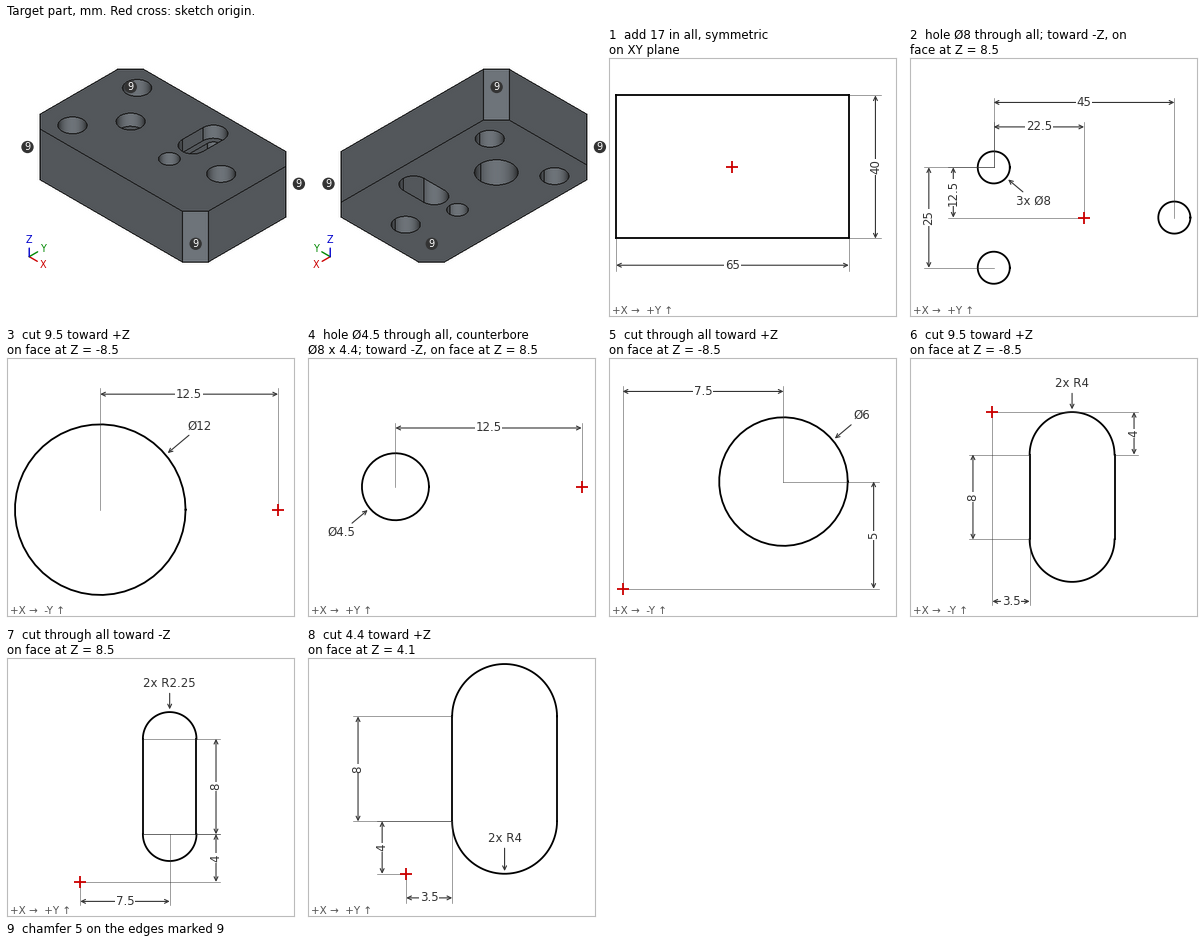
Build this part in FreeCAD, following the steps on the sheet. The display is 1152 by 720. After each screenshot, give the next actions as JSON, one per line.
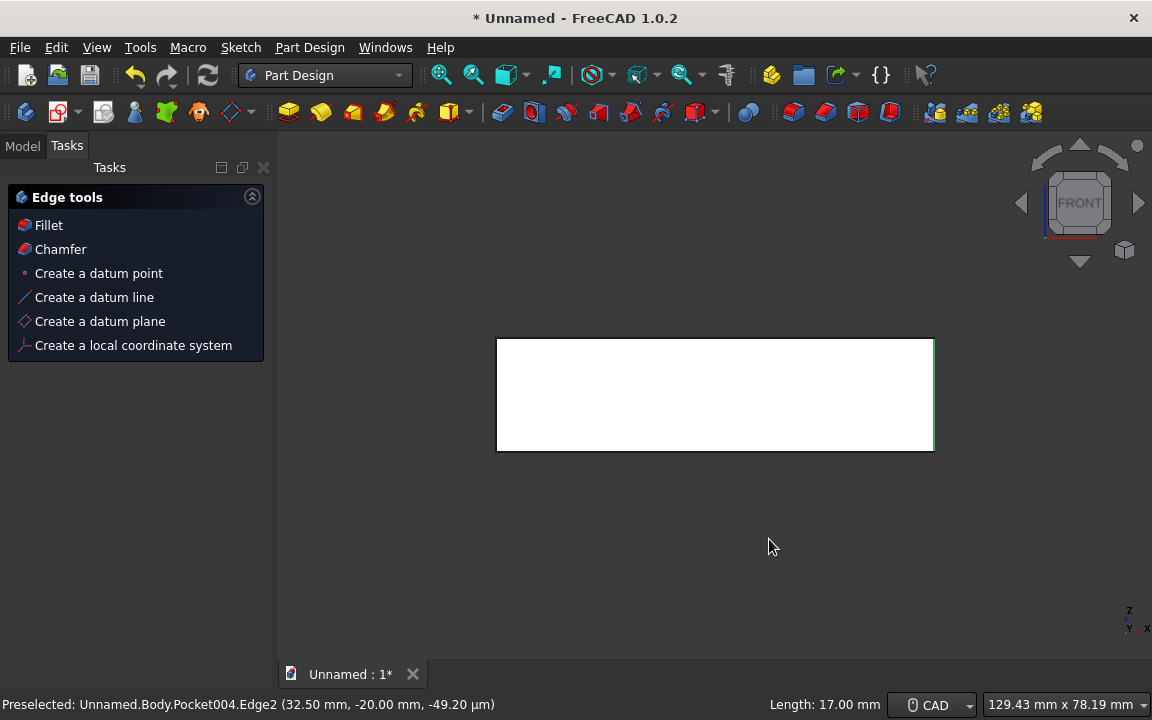
{"action": "left_click", "coordinate": [496, 394], "text": "ctrl"}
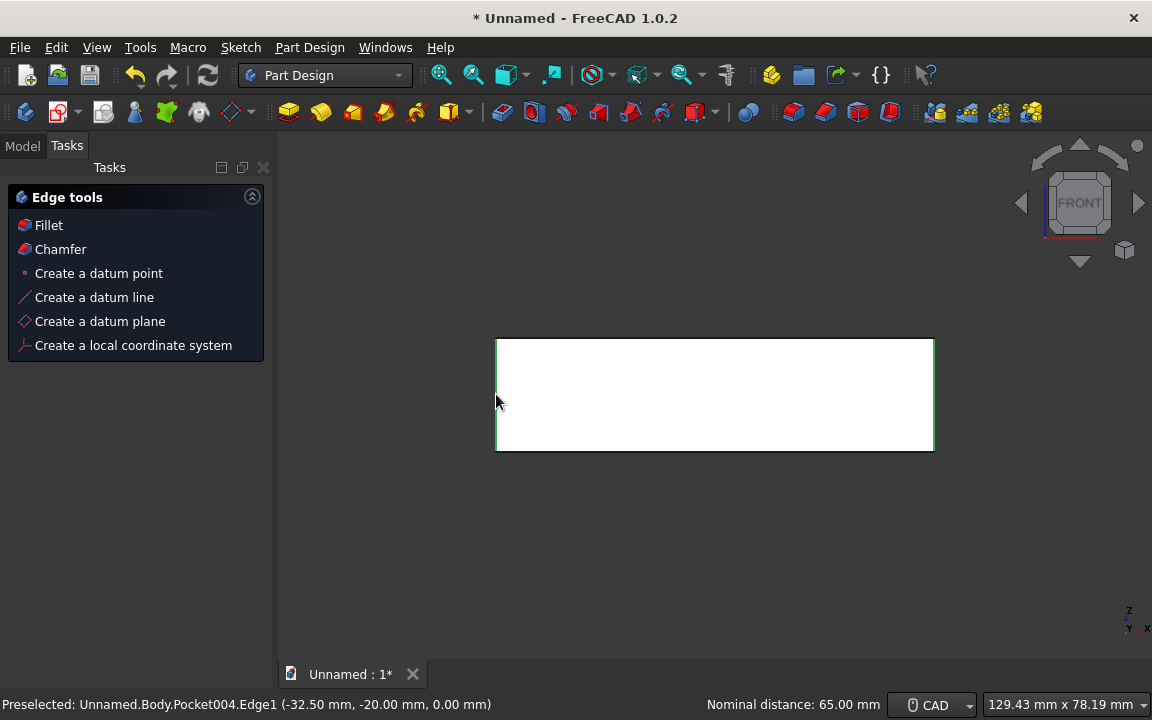
{"action": "key", "text": "3"}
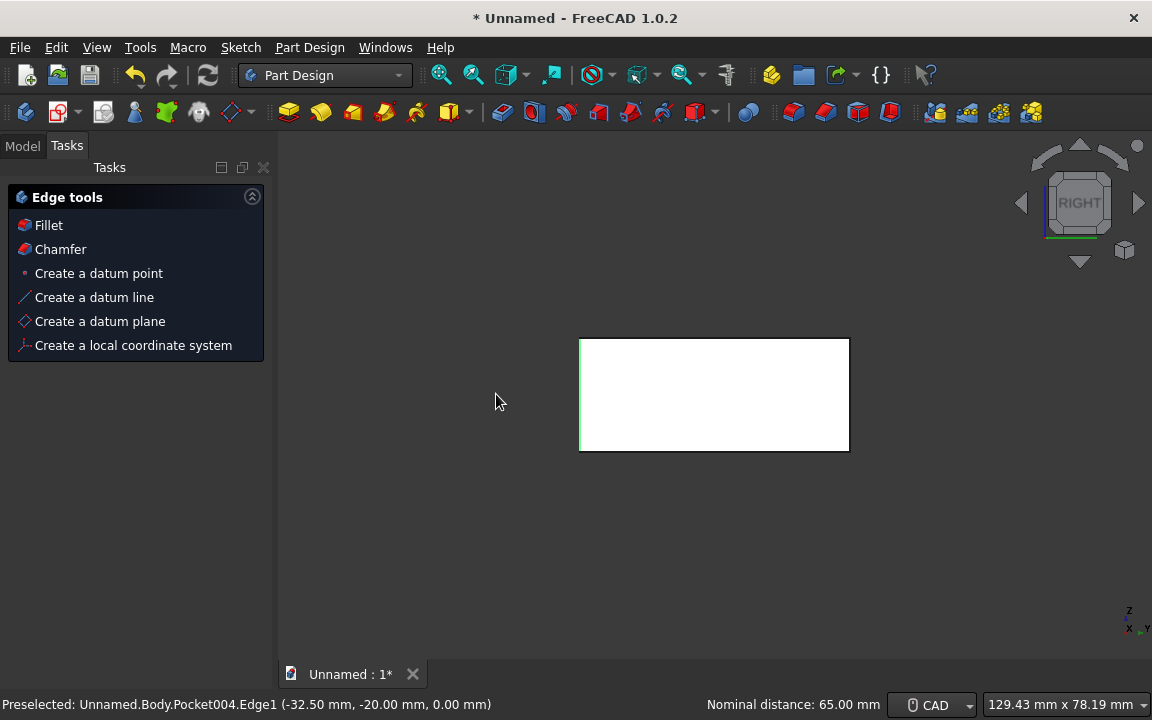
{"action": "left_click", "coordinate": [442, 76]}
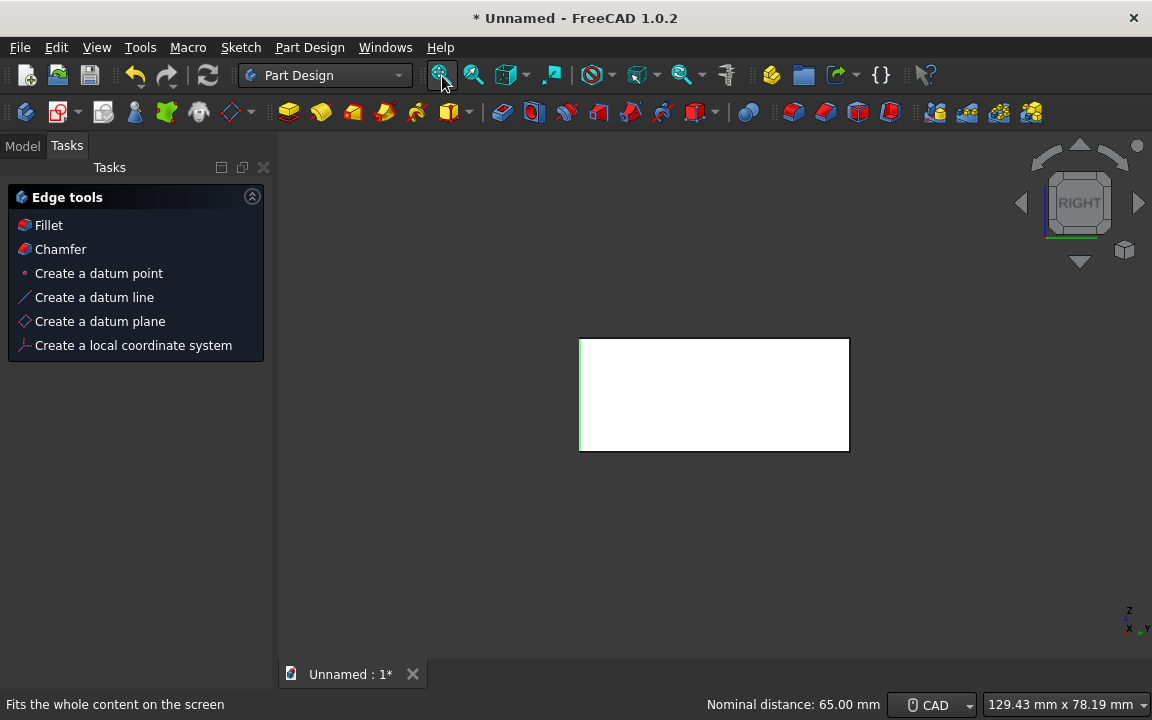
{"action": "left_click", "coordinate": [850, 394], "text": "ctrl"}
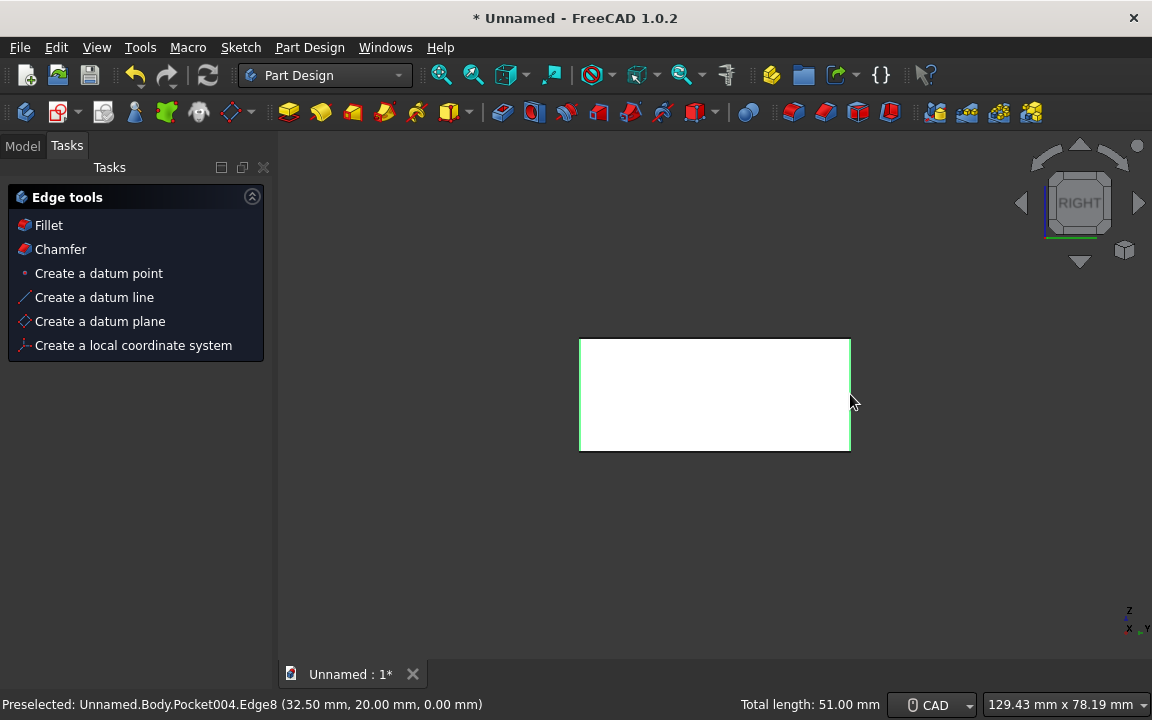
{"action": "key", "text": "5"}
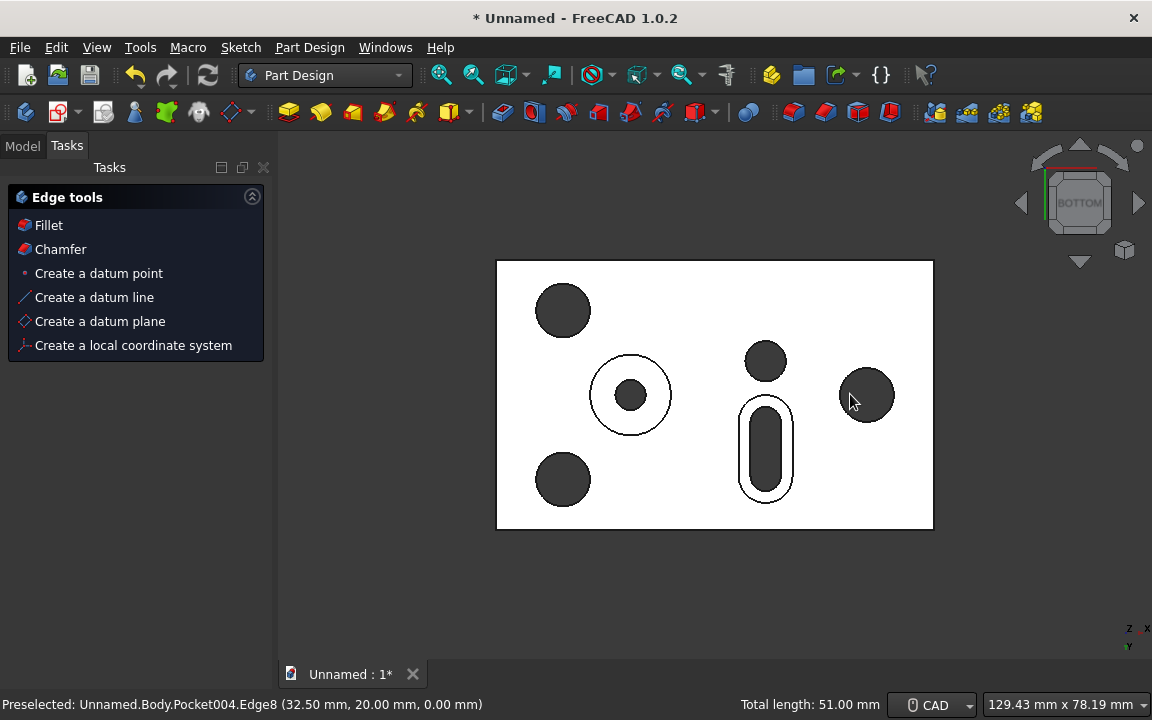
{"action": "key", "text": "4"}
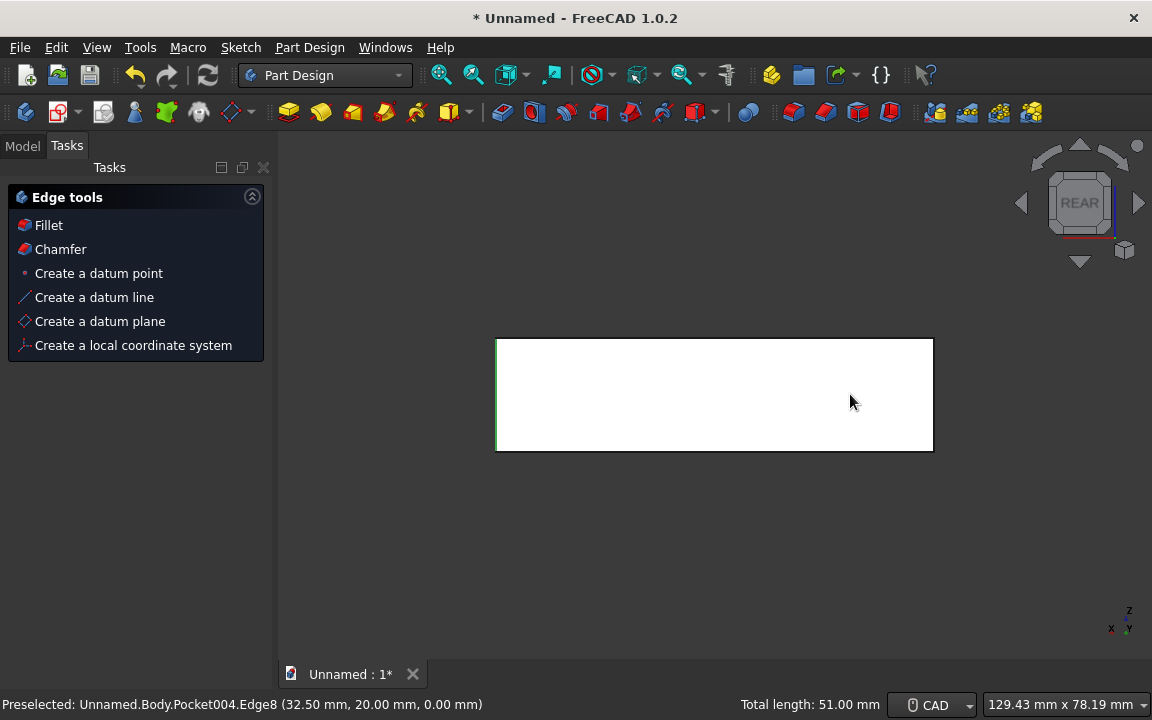
{"action": "left_click", "coordinate": [934, 394], "text": "ctrl"}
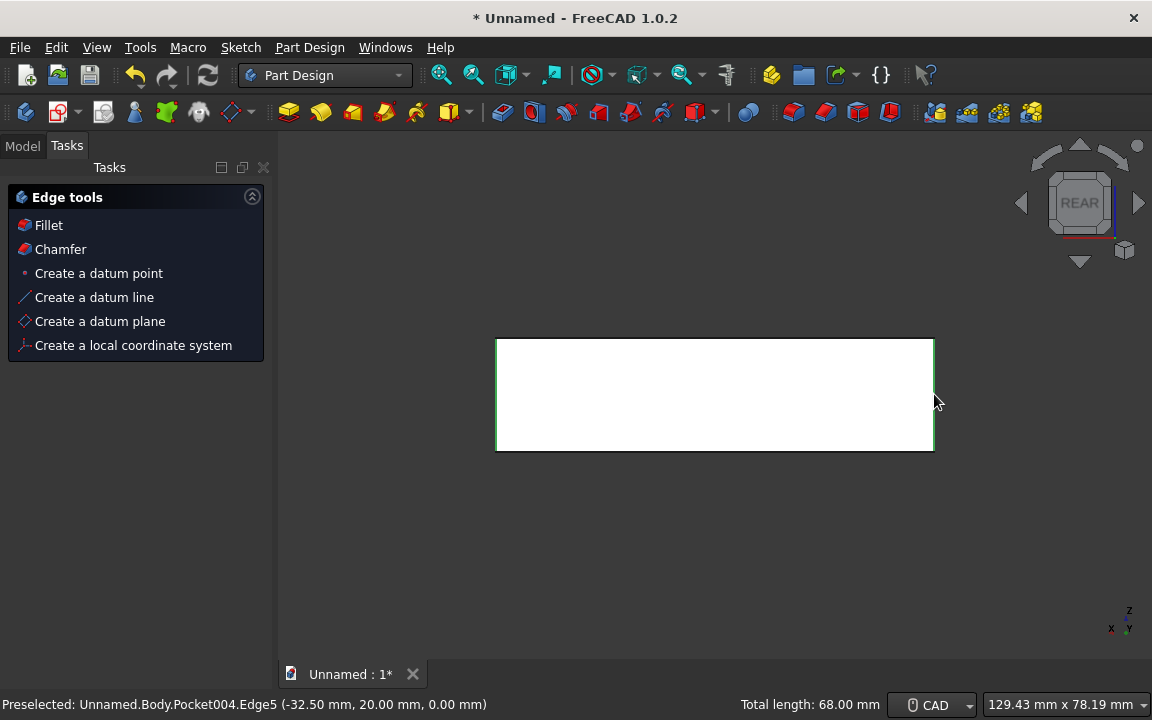
{"action": "left_click", "coordinate": [826, 112]}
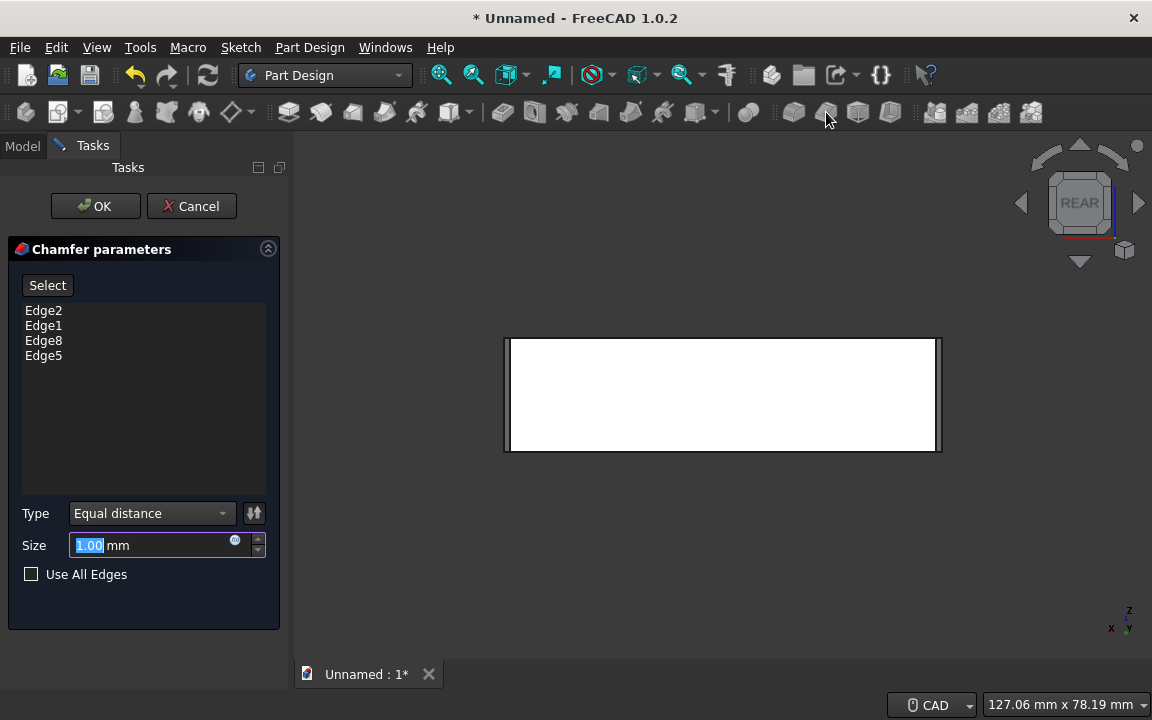
{"action": "type", "text": "5"}
{"action": "key", "text": "Tab"}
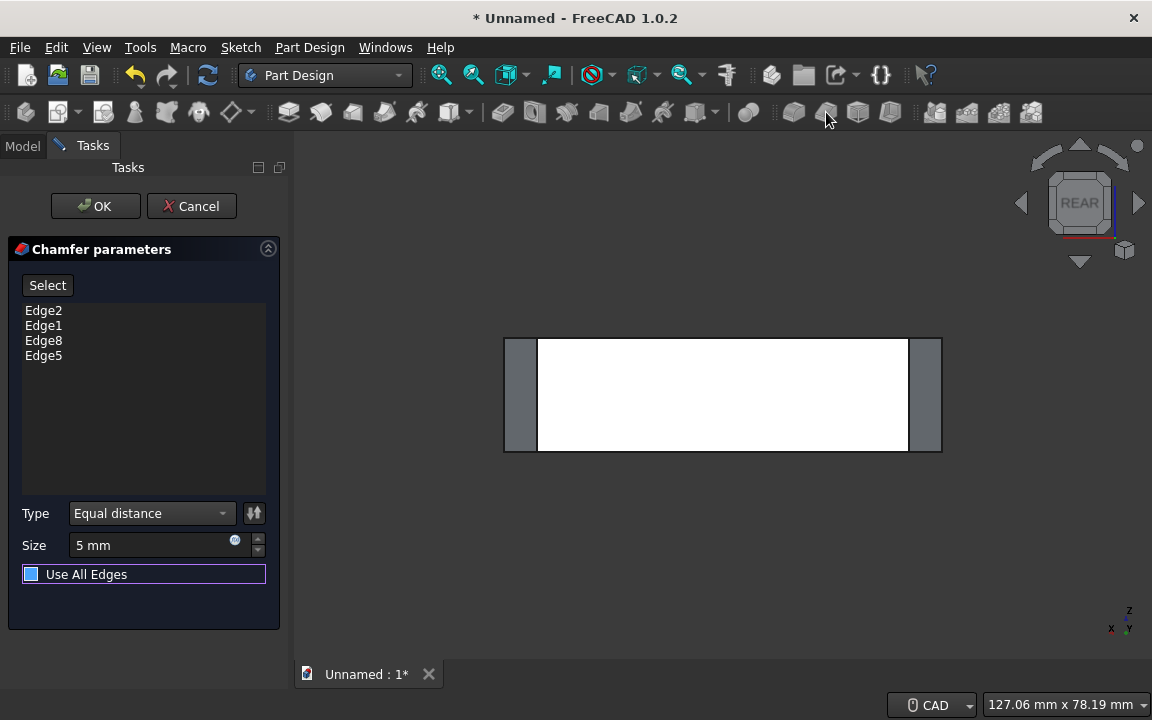
{"action": "left_click", "coordinate": [96, 206]}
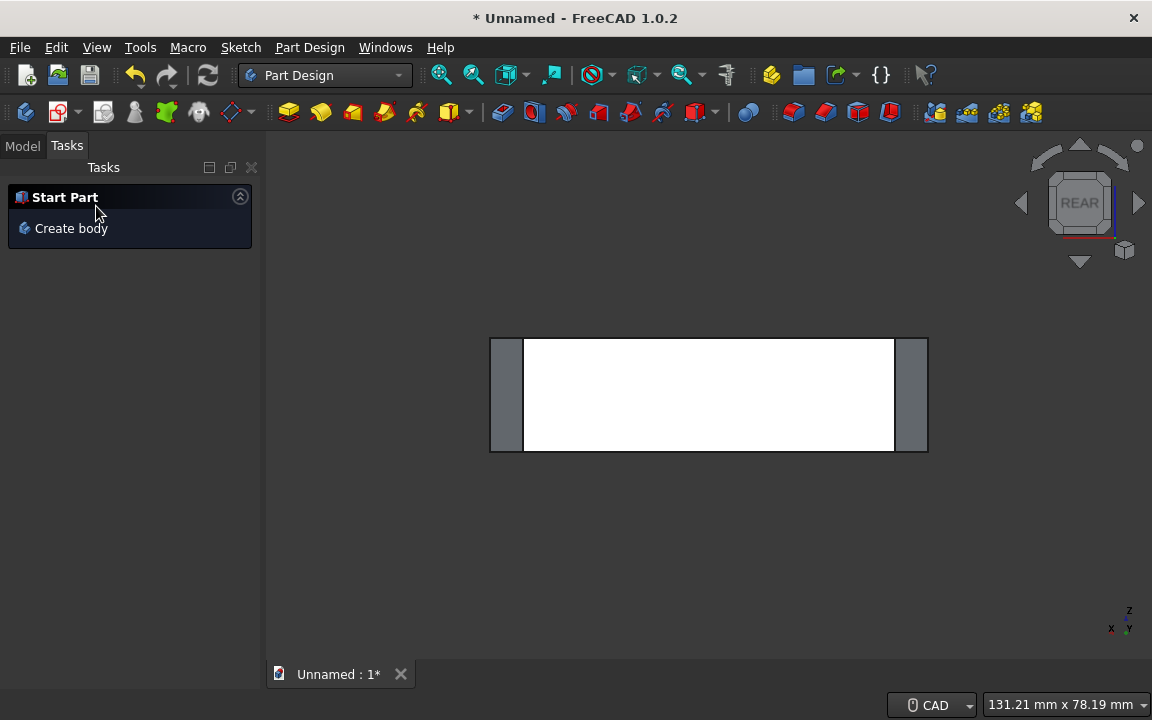
{"action": "key", "text": "0"}